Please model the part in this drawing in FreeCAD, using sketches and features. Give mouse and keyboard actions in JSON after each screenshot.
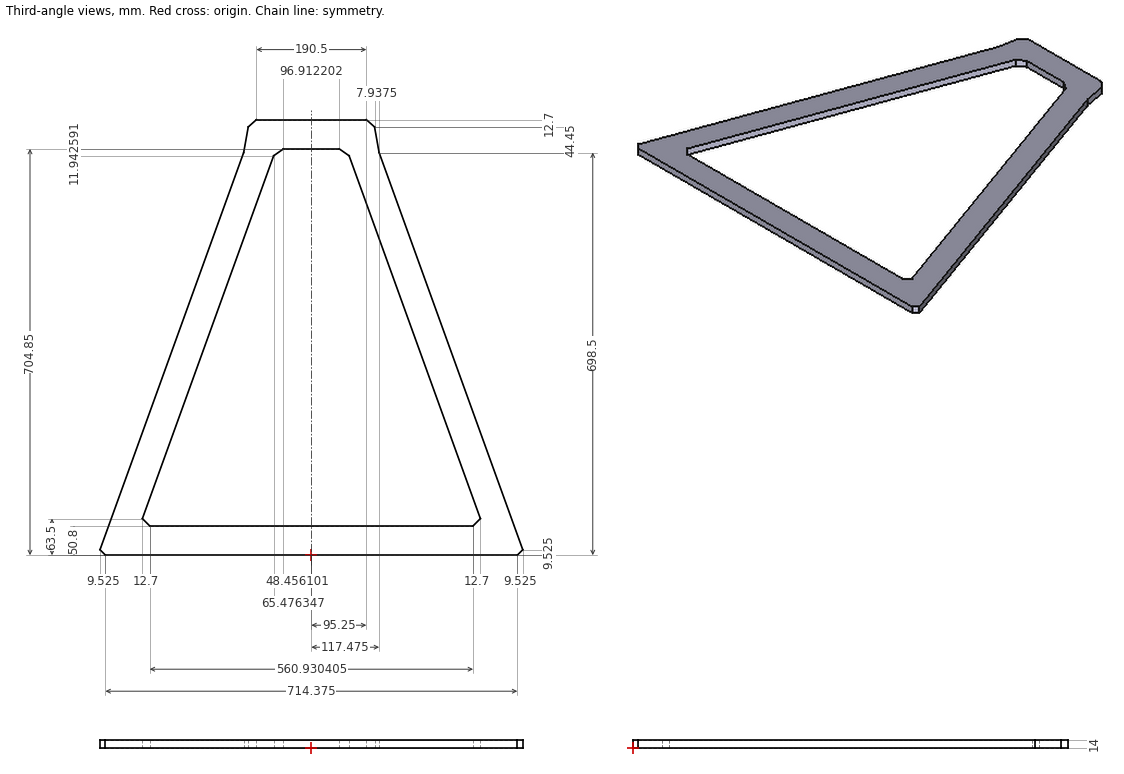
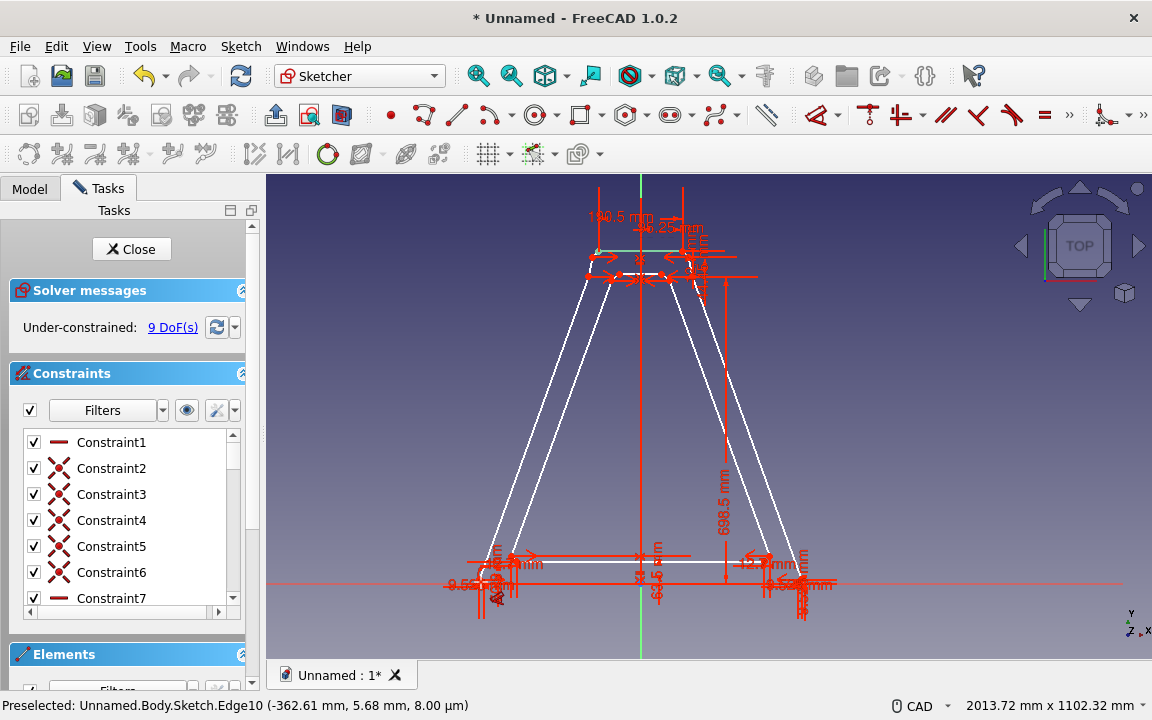
{"action": "left_click", "coordinate": [578, 584]}
{"action": "left_click", "coordinate": [568, 618]}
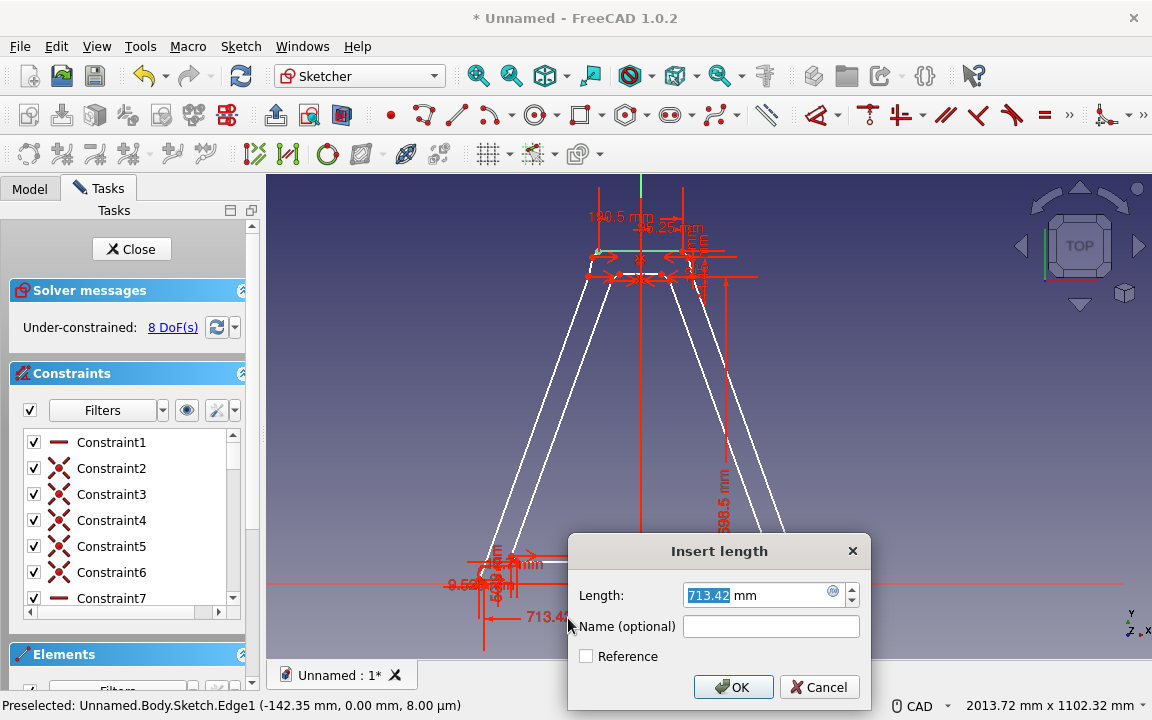
{"action": "type", "text": "714.375"}
{"action": "key", "text": "Return"}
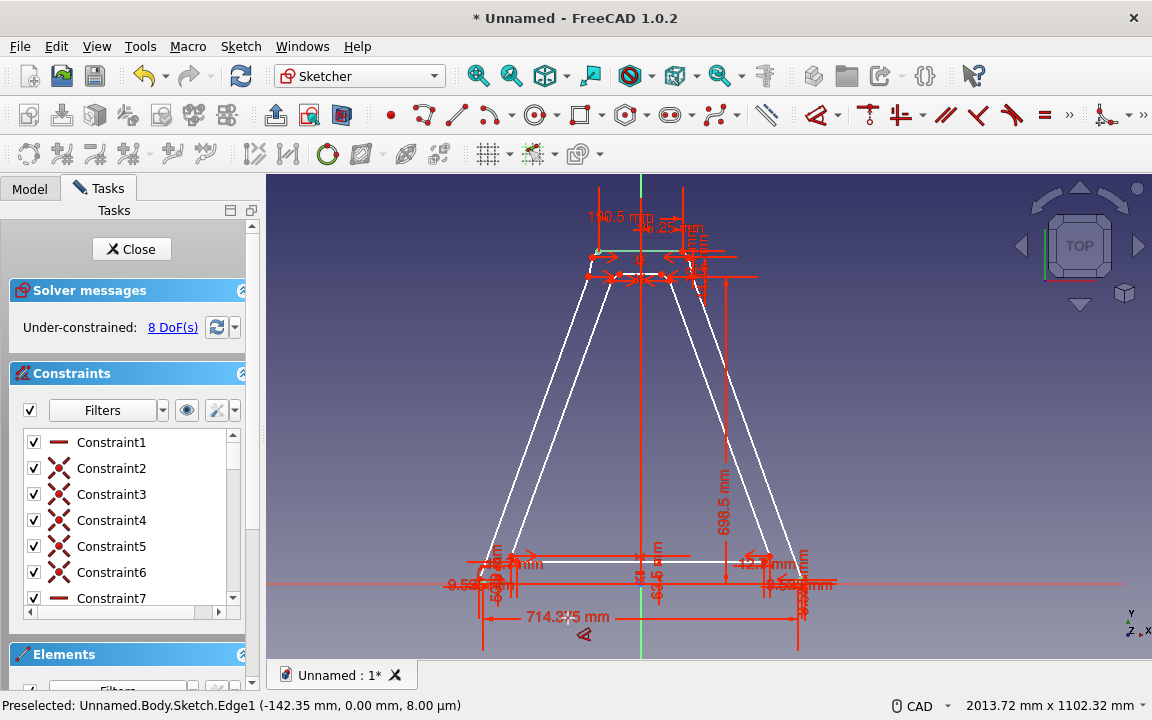
{"action": "scroll", "coordinate": [619, 274], "scroll_direction": "up", "scroll_amount": 2}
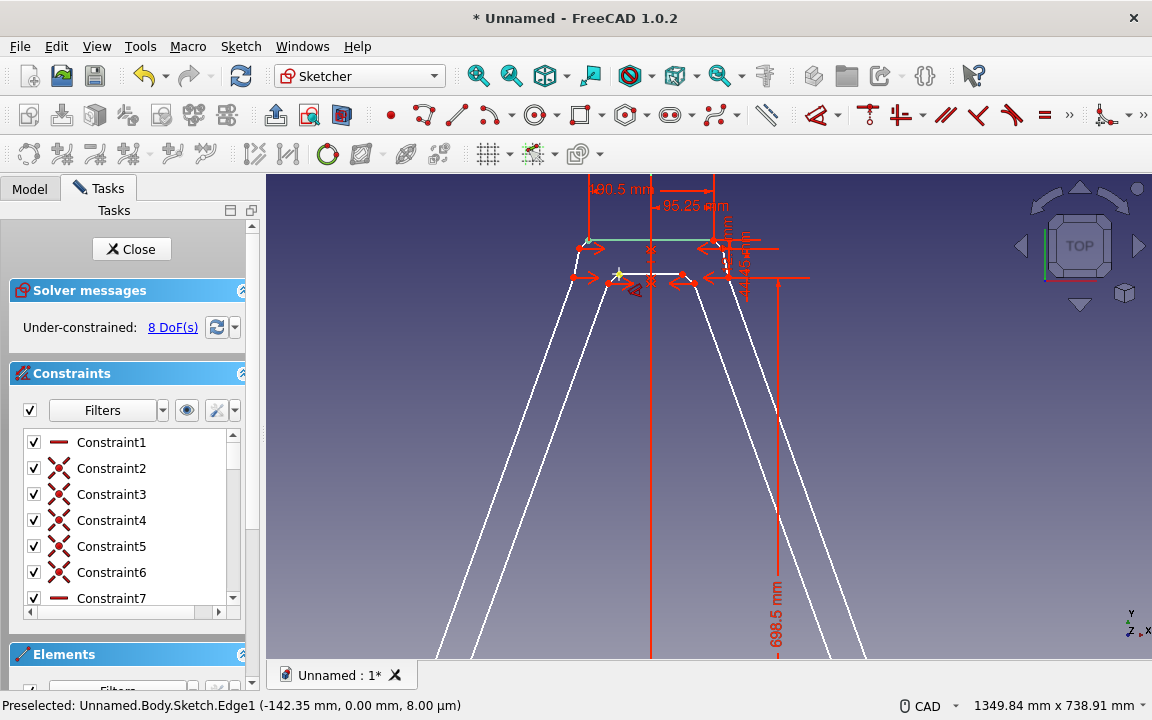
{"action": "left_click", "coordinate": [619, 274]}
{"action": "left_click", "coordinate": [585, 453]}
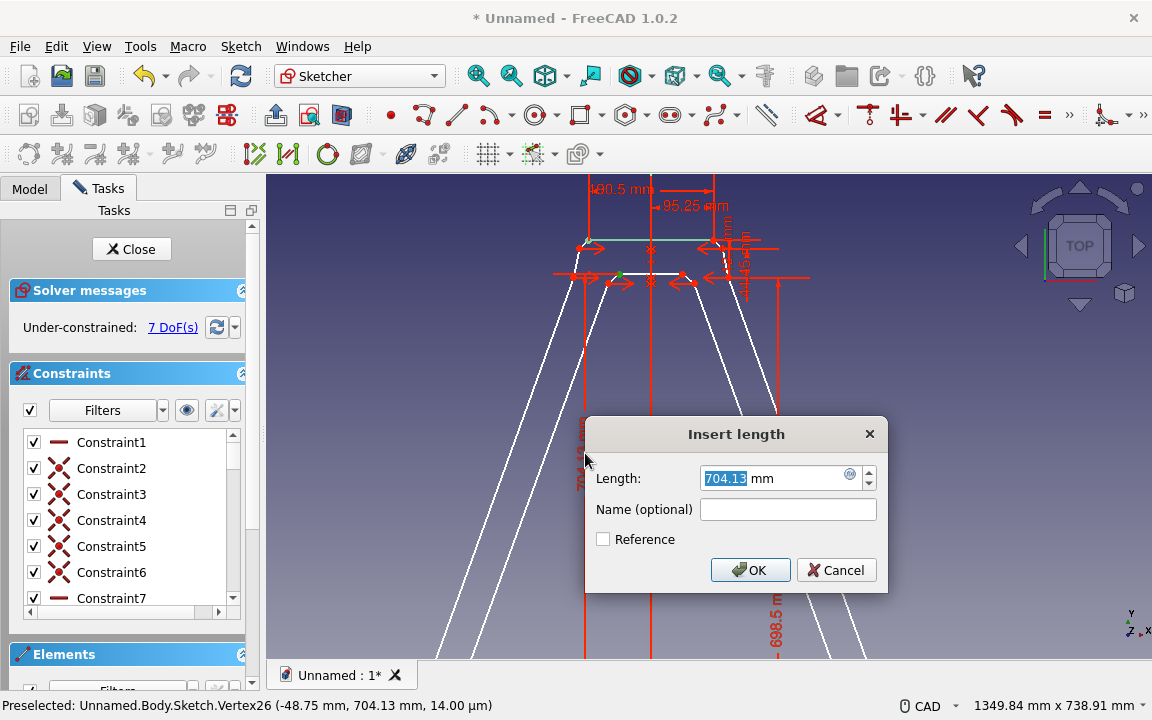
{"action": "type", "text": "704.85"}
{"action": "key", "text": "Return"}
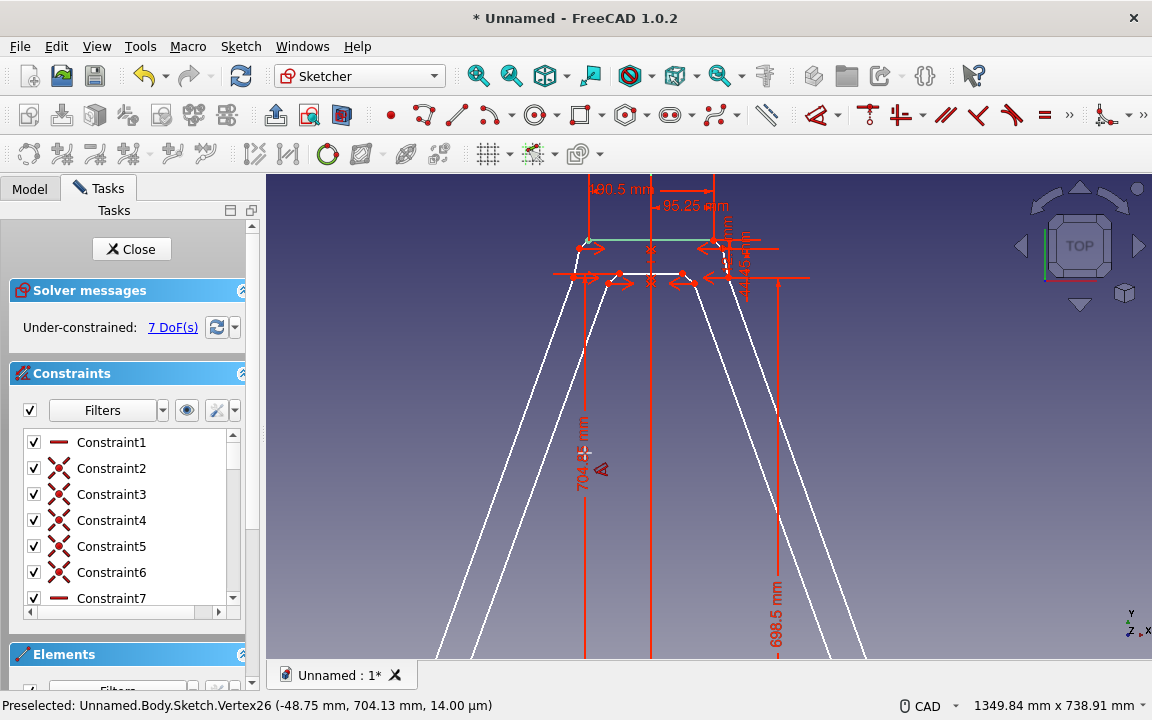
{"action": "scroll", "coordinate": [726, 266], "scroll_direction": "up", "scroll_amount": 11}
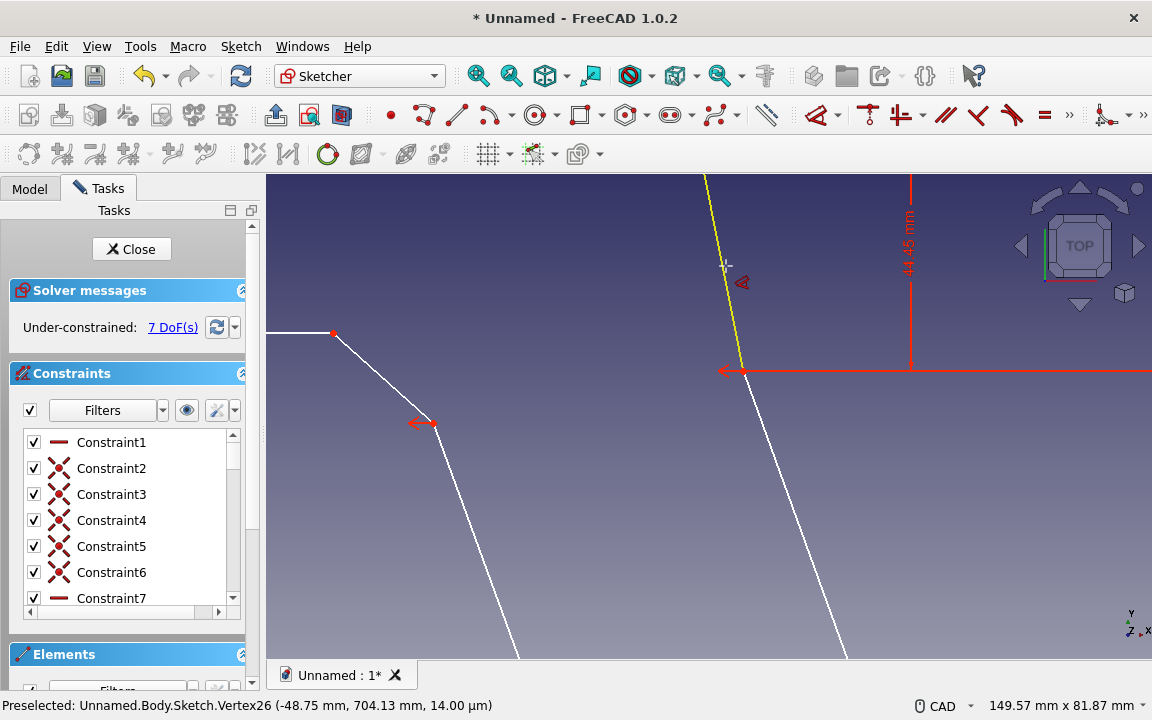
{"action": "left_click", "coordinate": [722, 266]}
{"action": "left_click", "coordinate": [717, 405]}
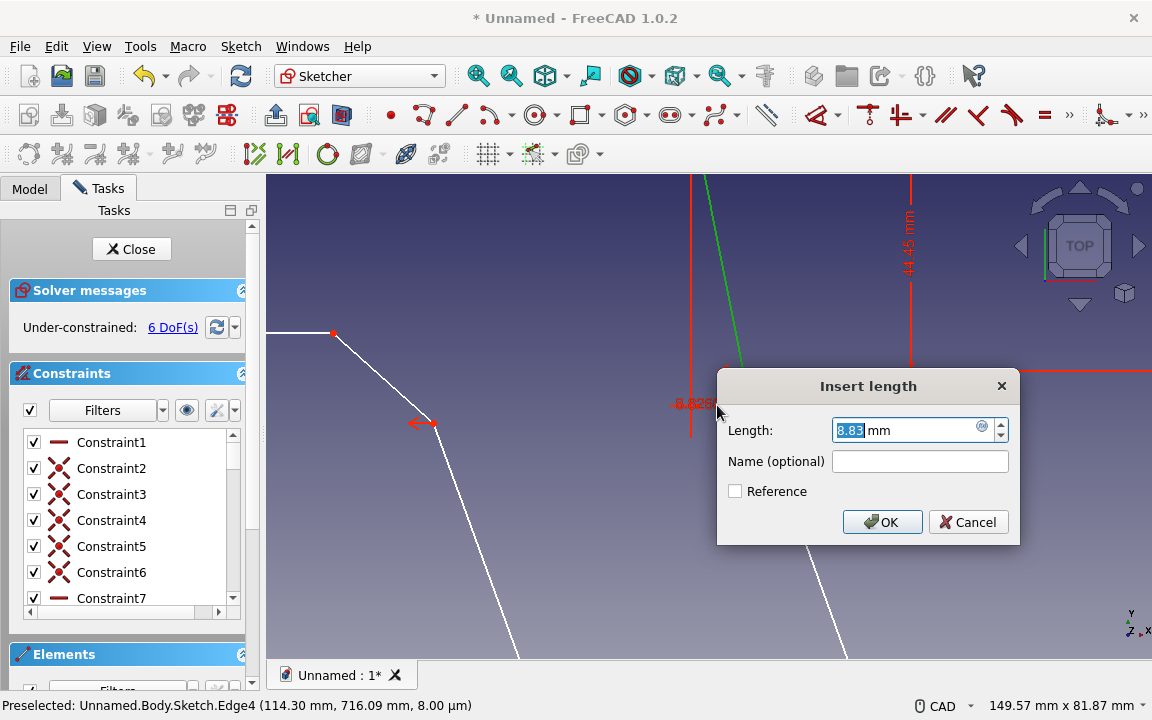
{"action": "type", "text": "7.9375"}
{"action": "key", "text": "Return"}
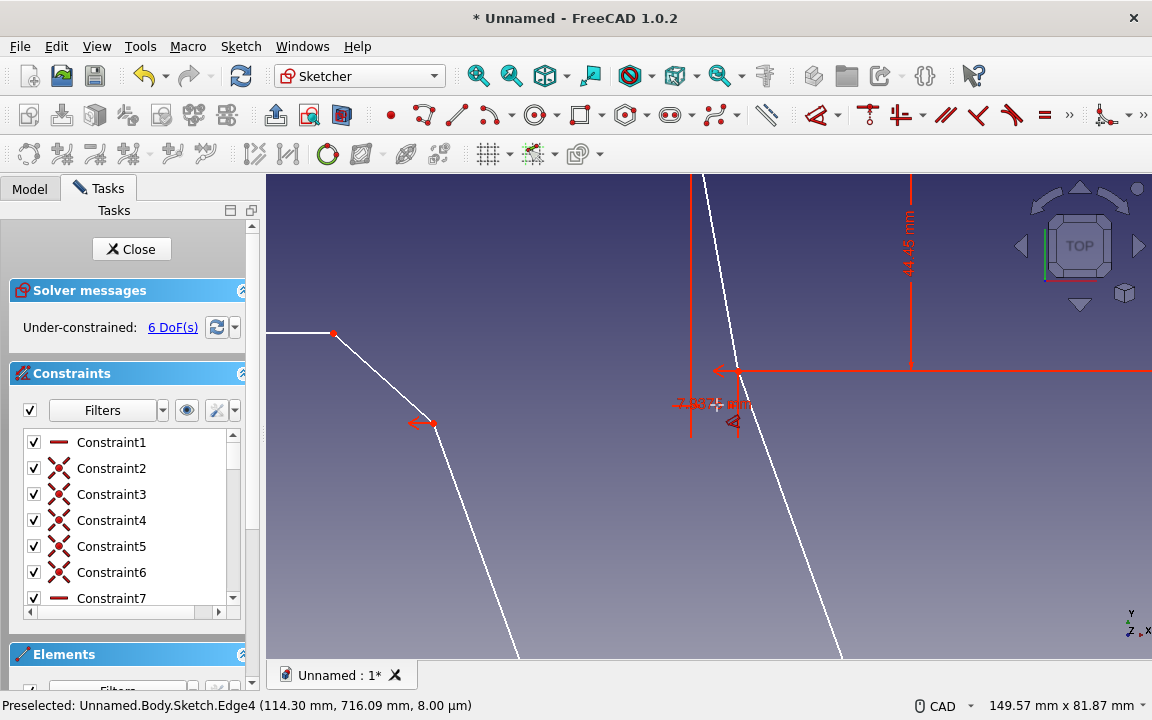
{"action": "scroll", "coordinate": [688, 268], "scroll_direction": "down", "scroll_amount": 13}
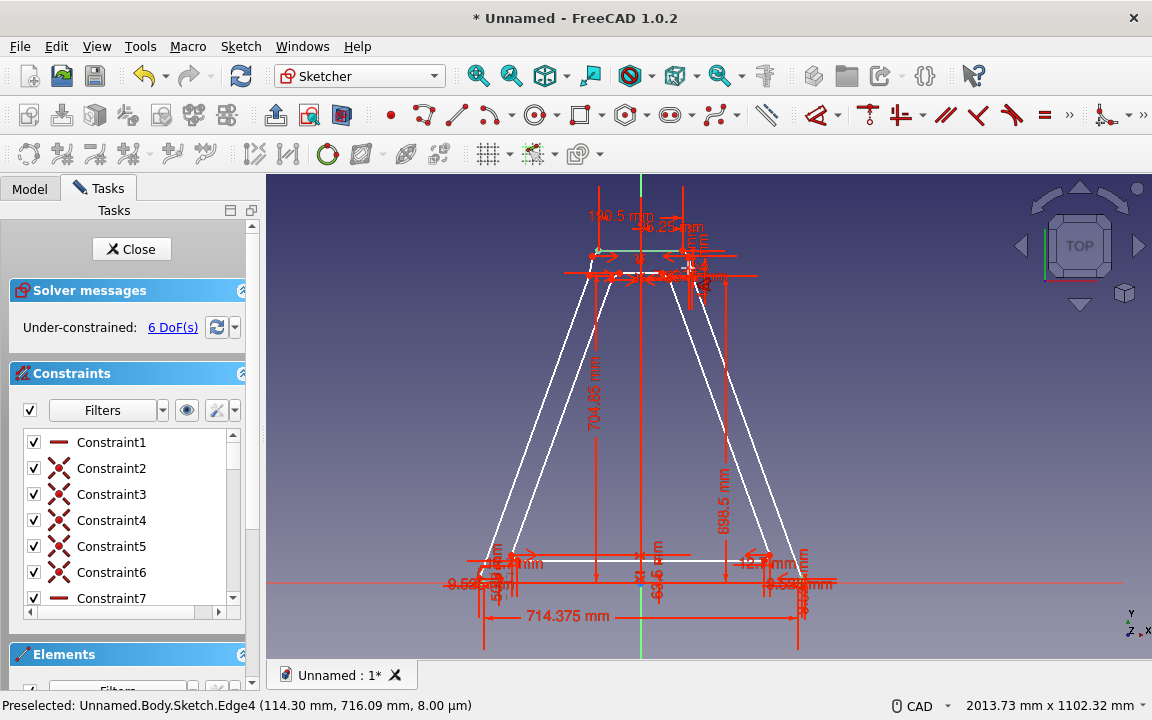
{"action": "left_click", "coordinate": [692, 276]}
{"action": "left_click", "coordinate": [666, 617]}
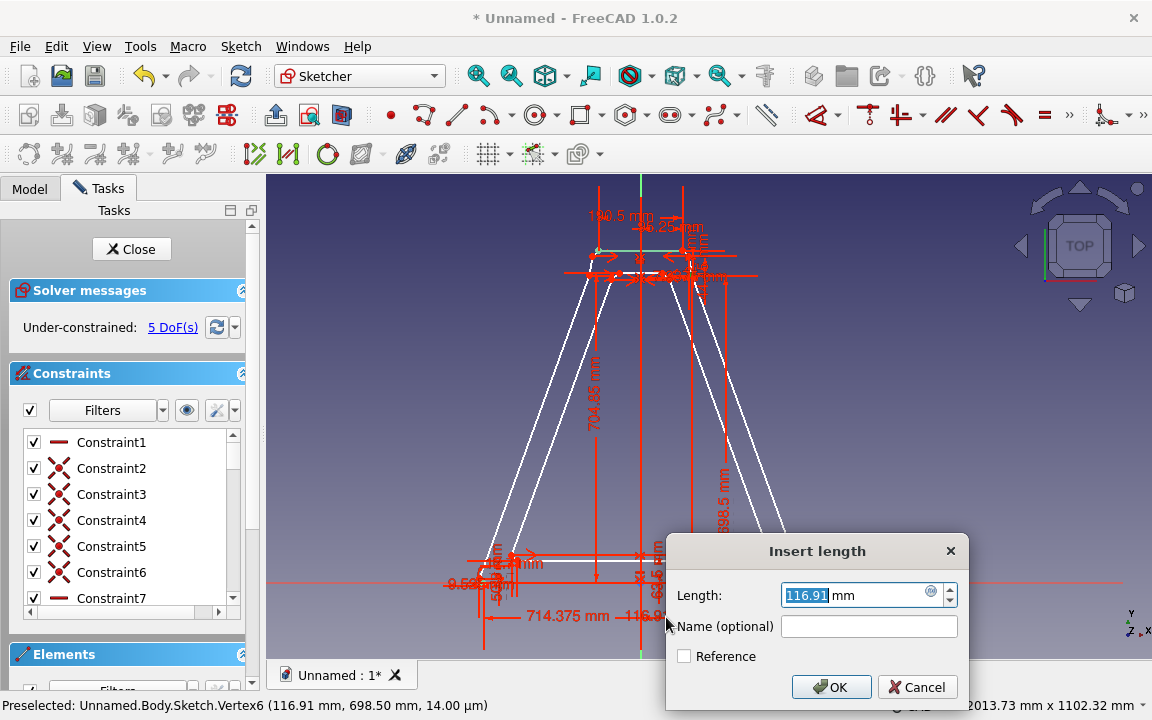
{"action": "type", "text": "117.475"}
{"action": "key", "text": "Return"}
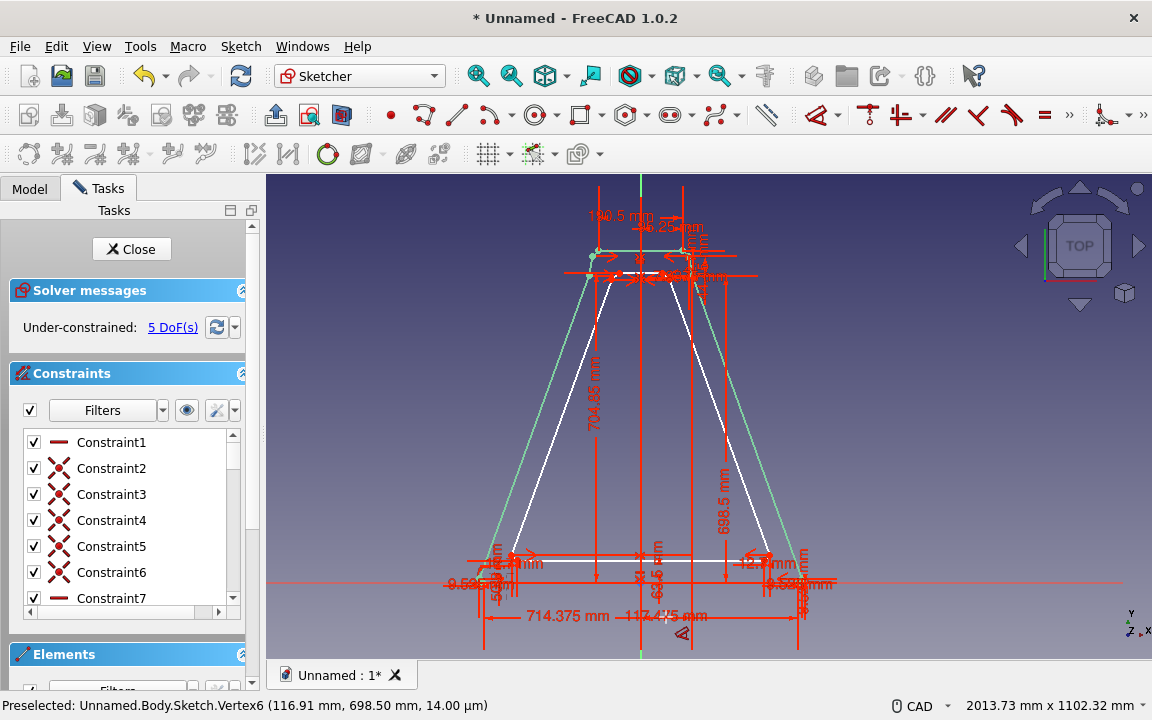
{"action": "left_click", "coordinate": [641, 273]}
{"action": "left_click", "coordinate": [626, 307]}